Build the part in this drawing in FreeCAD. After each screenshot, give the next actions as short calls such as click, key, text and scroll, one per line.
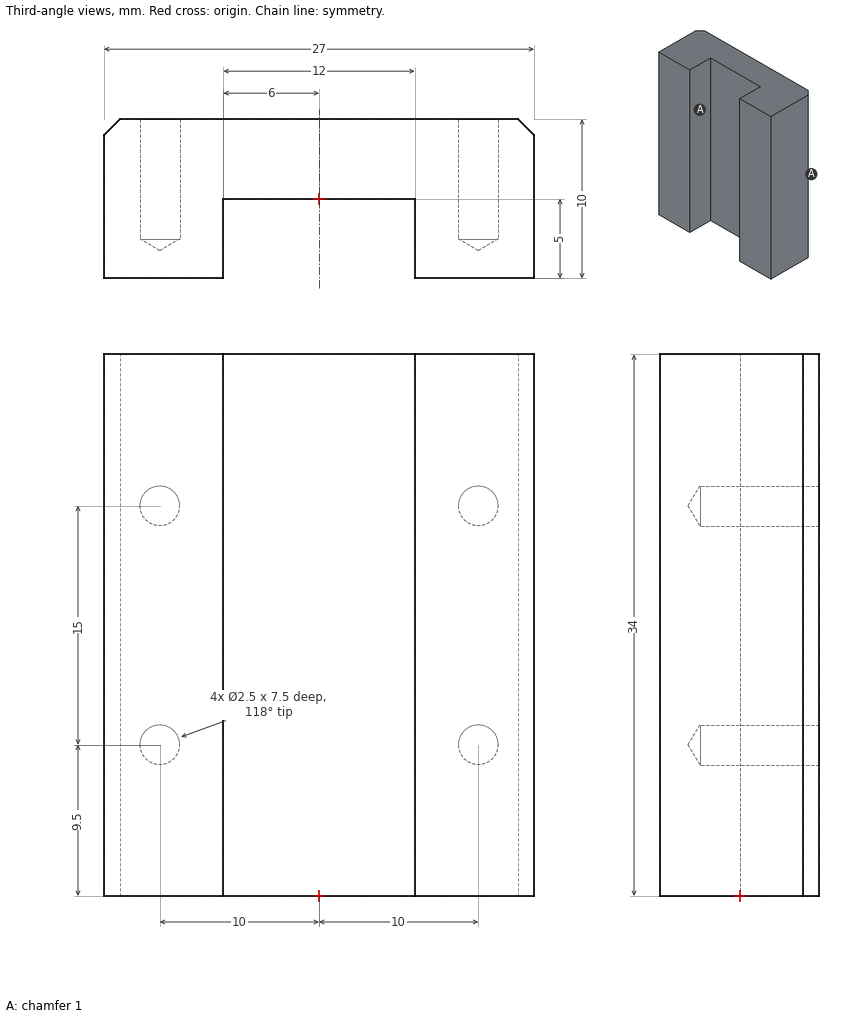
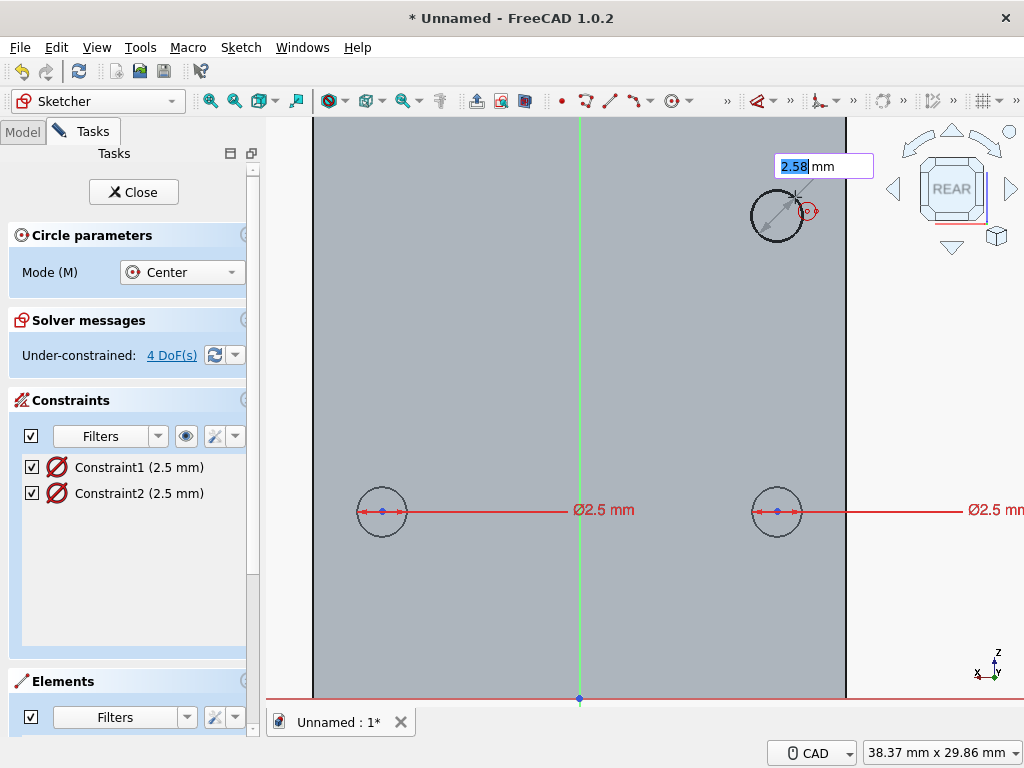
text(2.5)
key(Return)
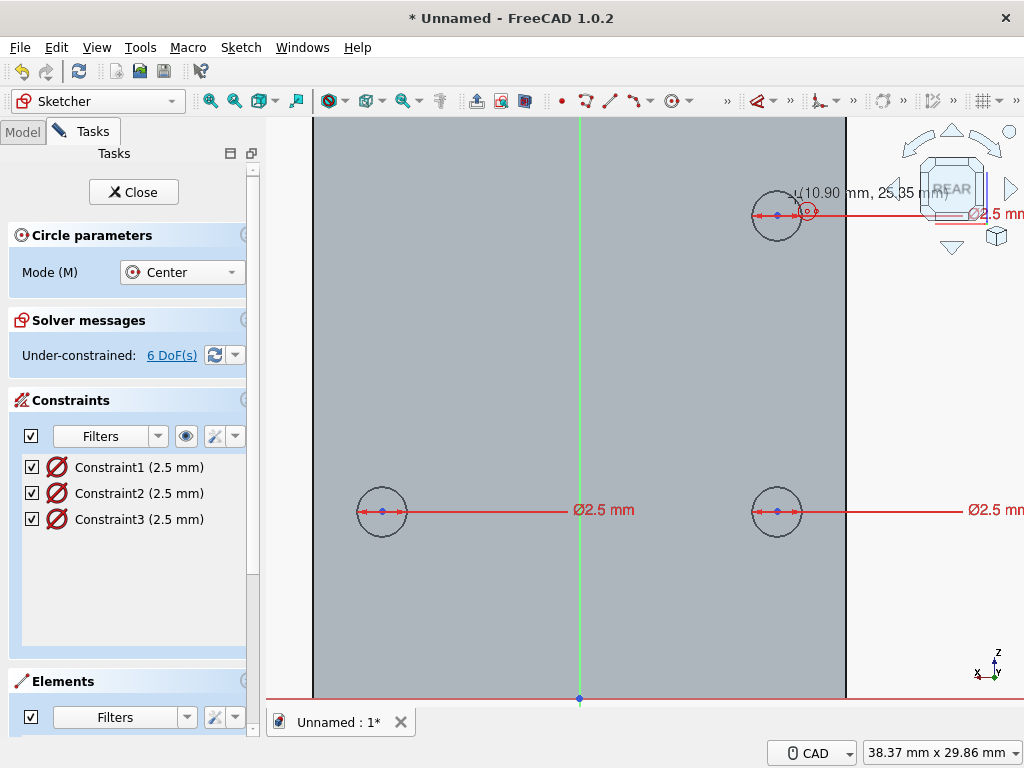
click(382, 215)
move(400, 197)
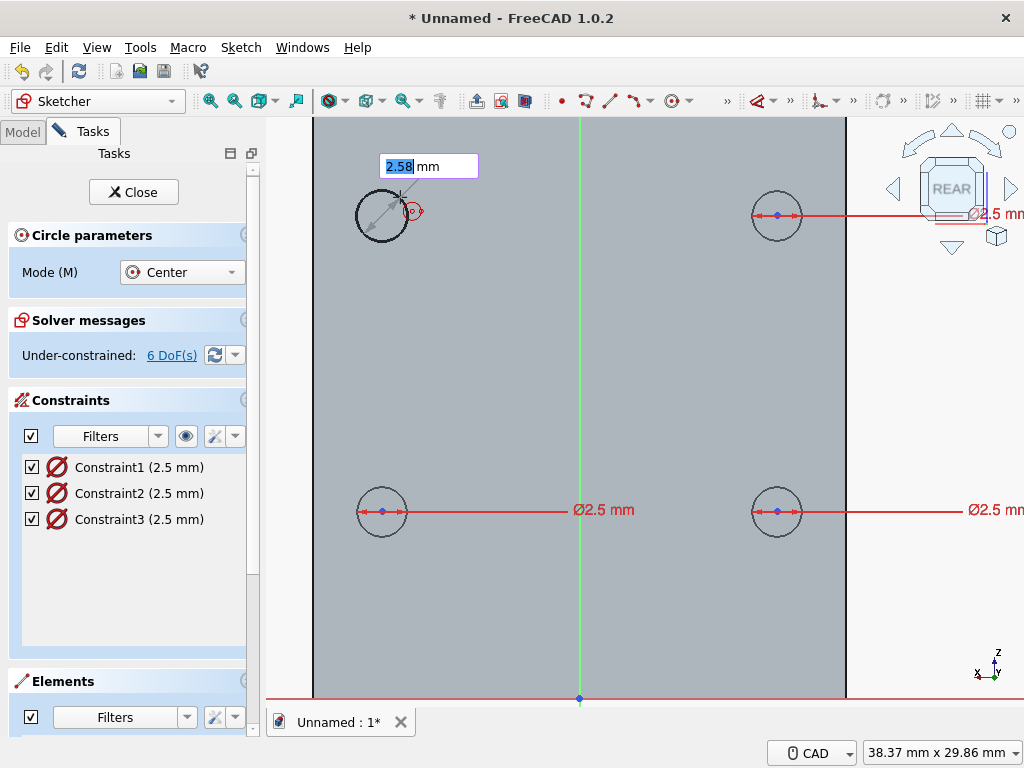
text(2.5)
key(Return)
key(Escape)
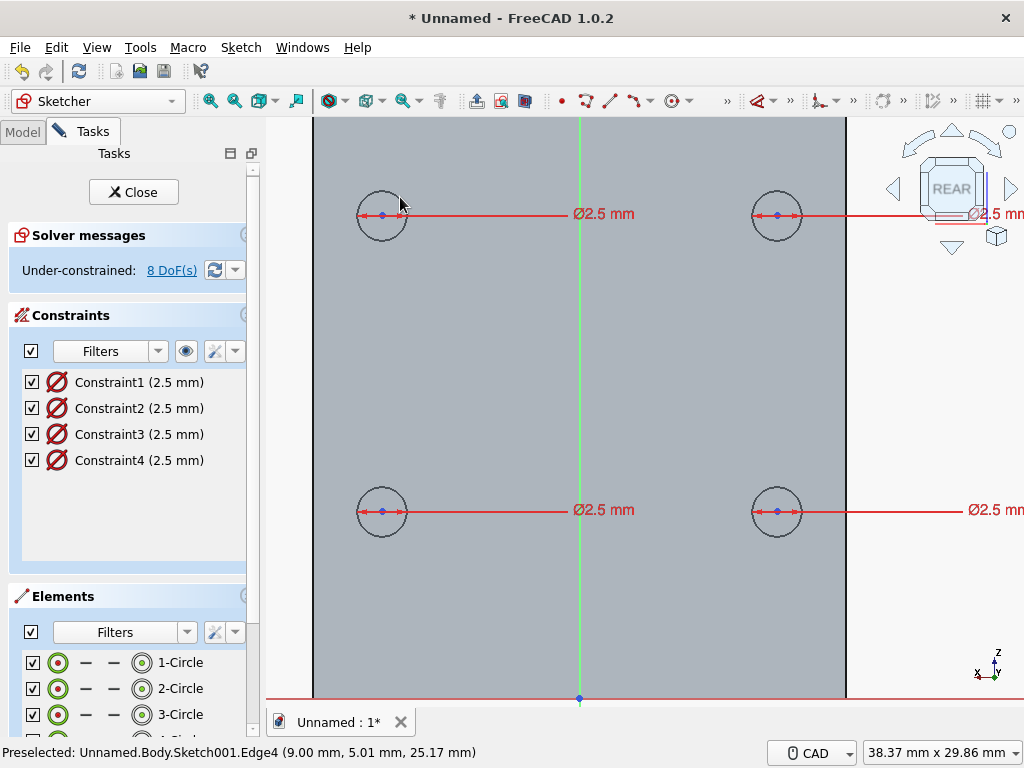
click(777, 512)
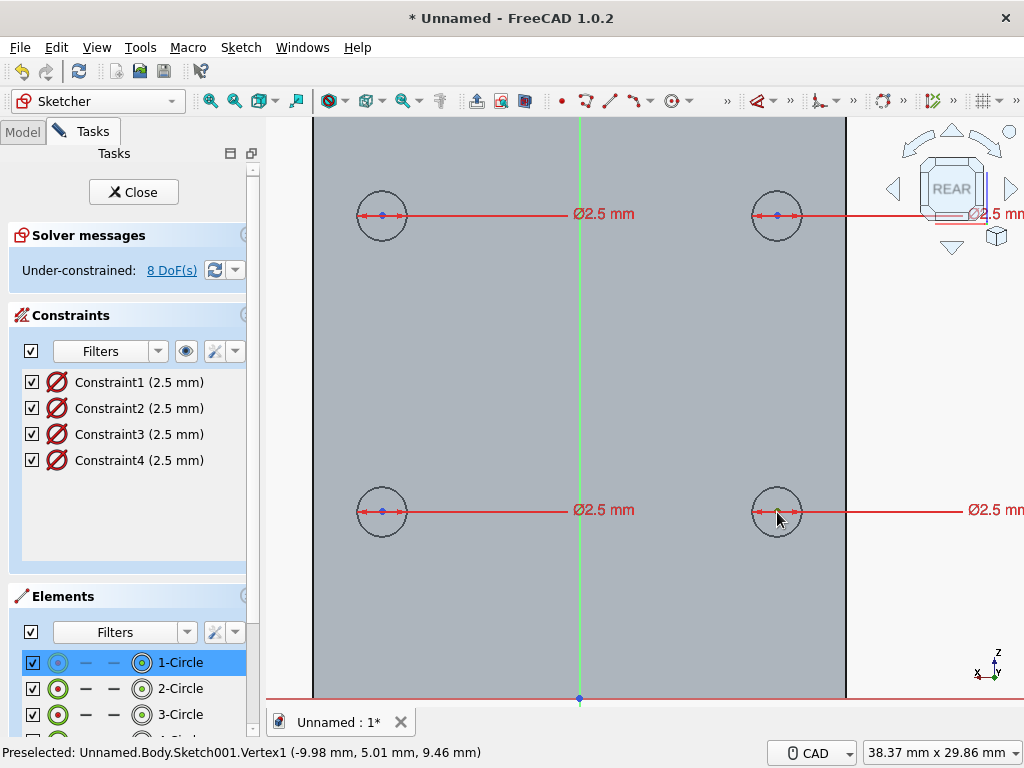
click(382, 512)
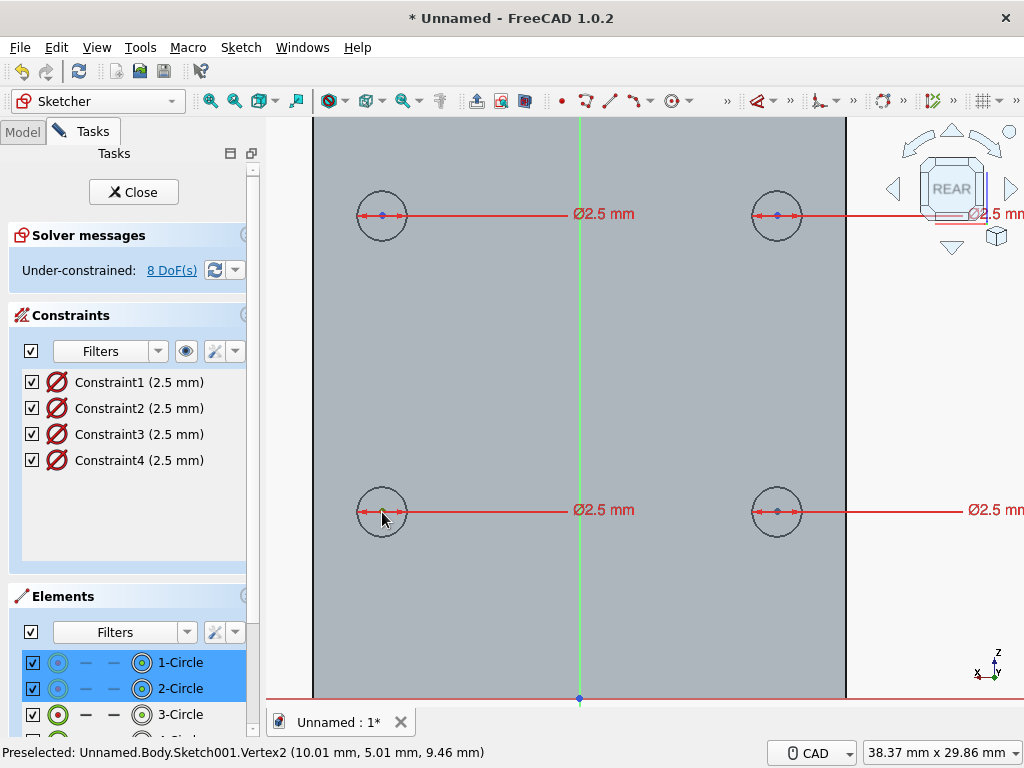
key(h)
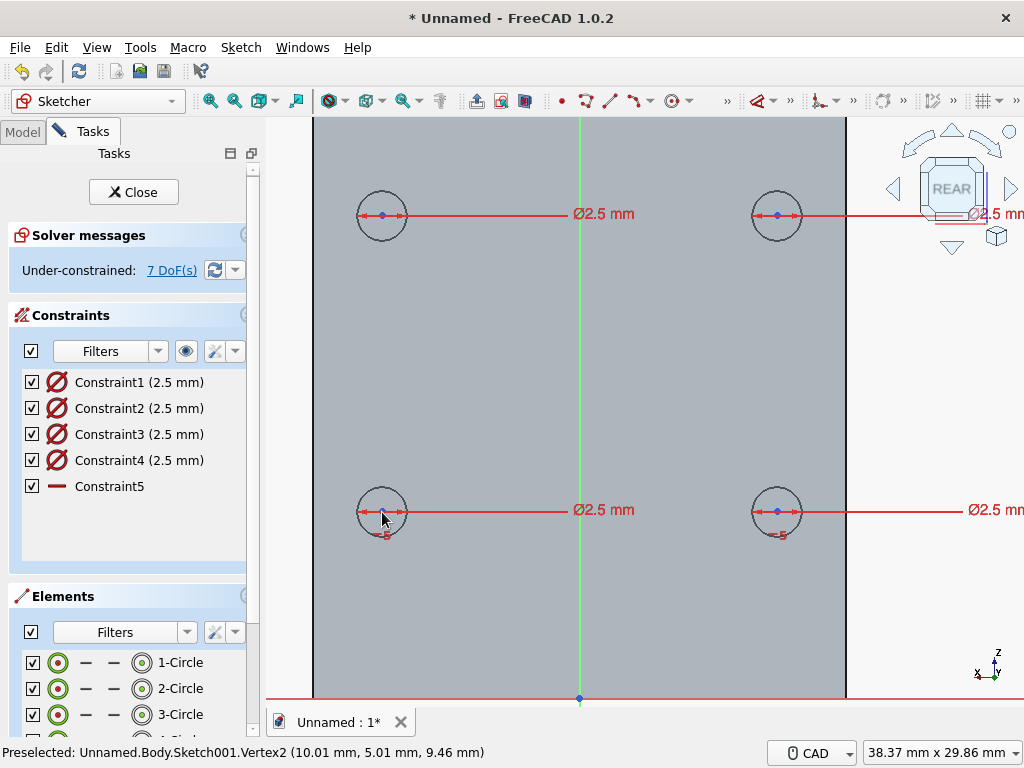
click(777, 512)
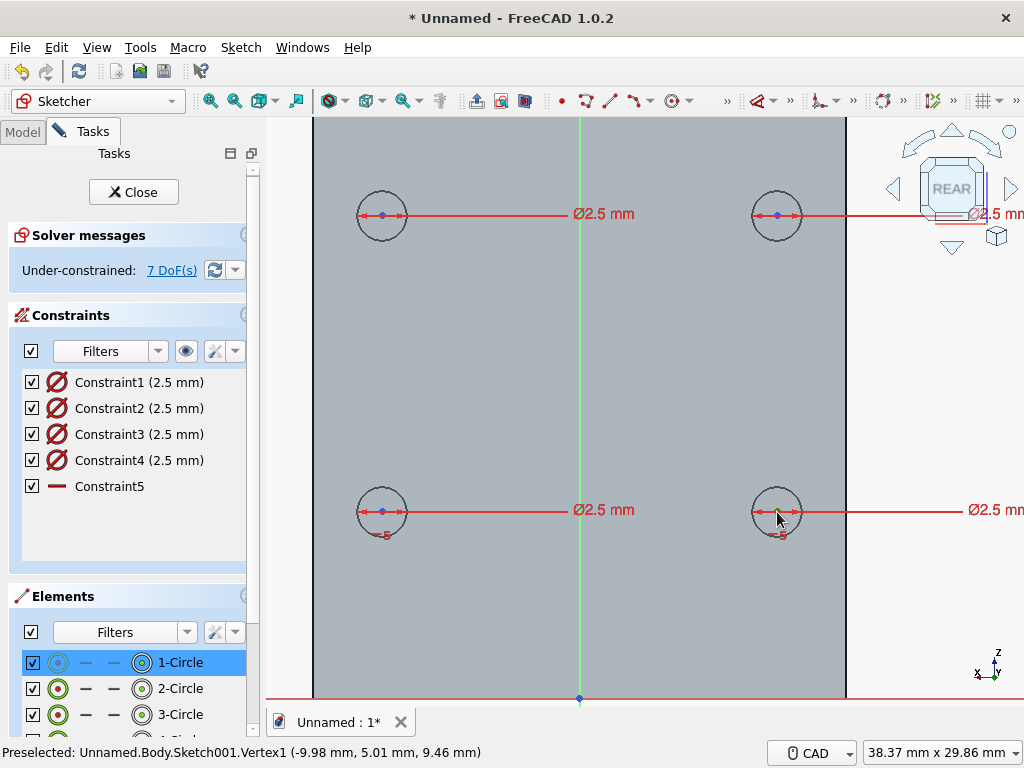
click(777, 216)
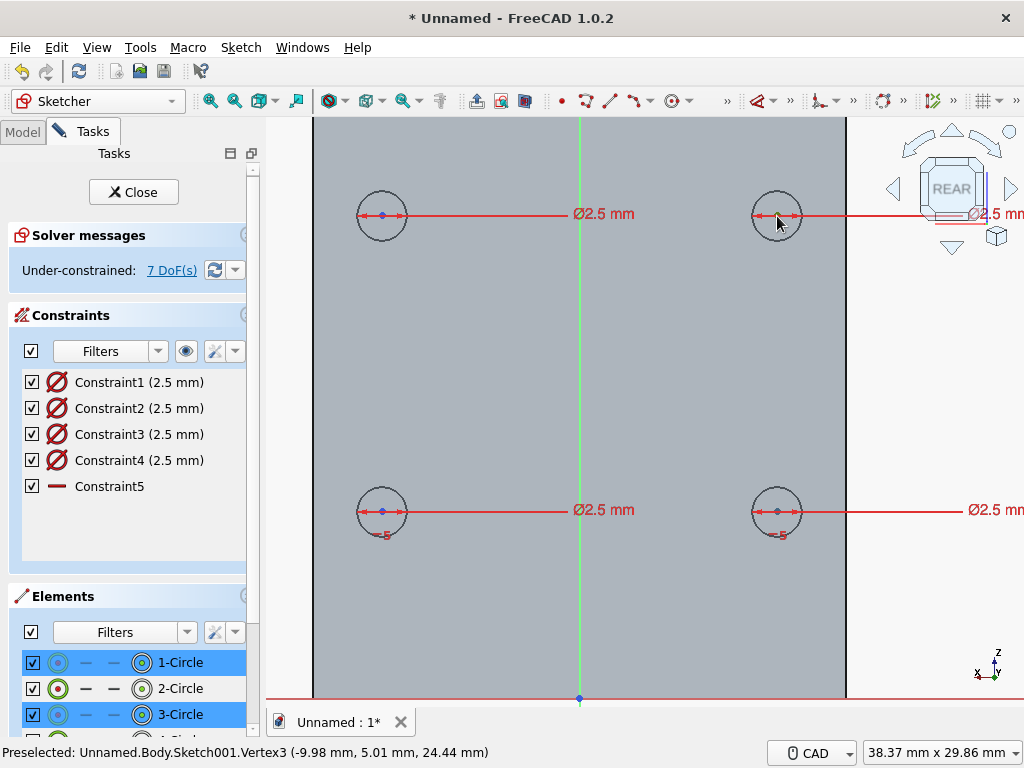
key(v)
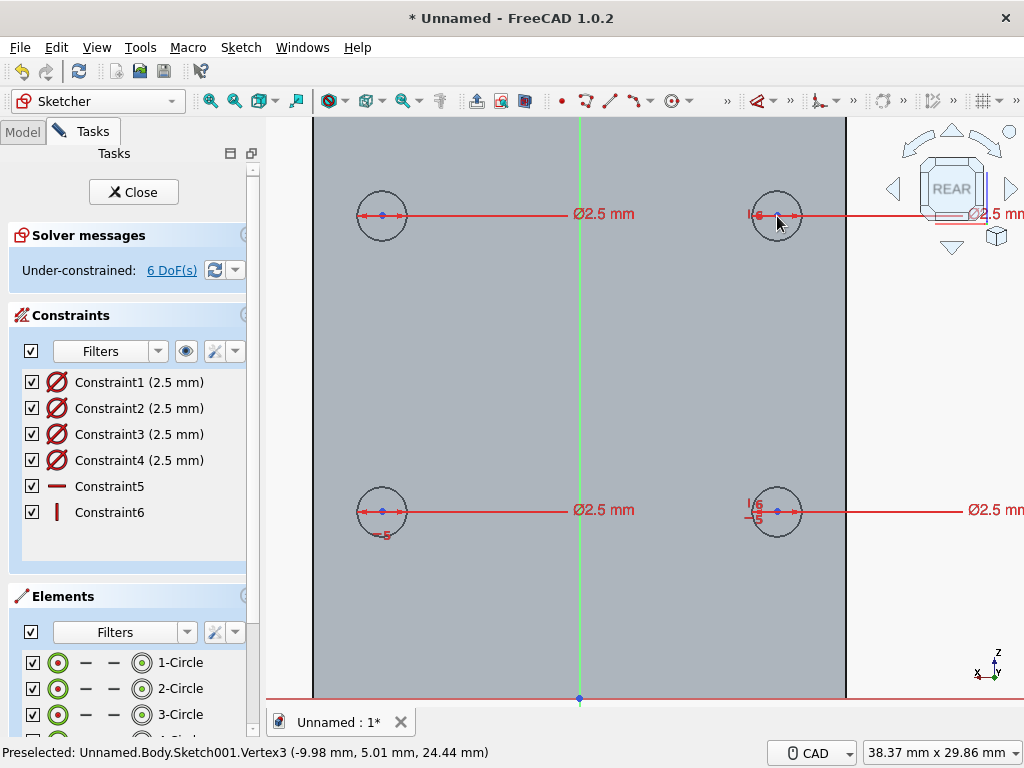
click(382, 512)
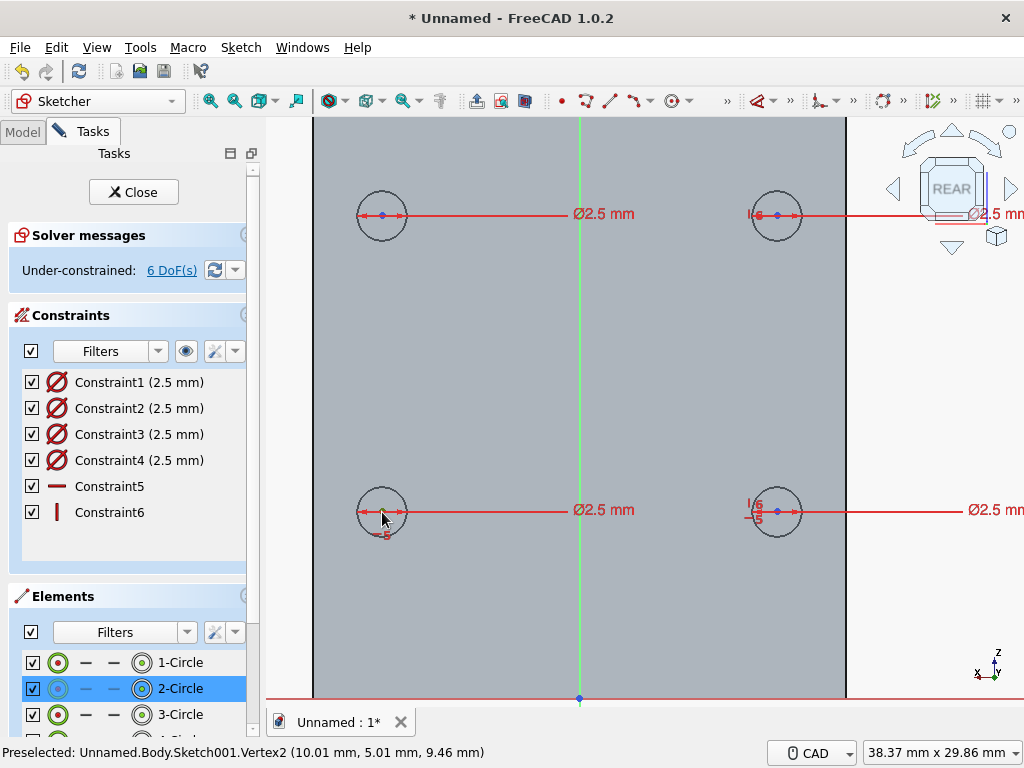
click(382, 216)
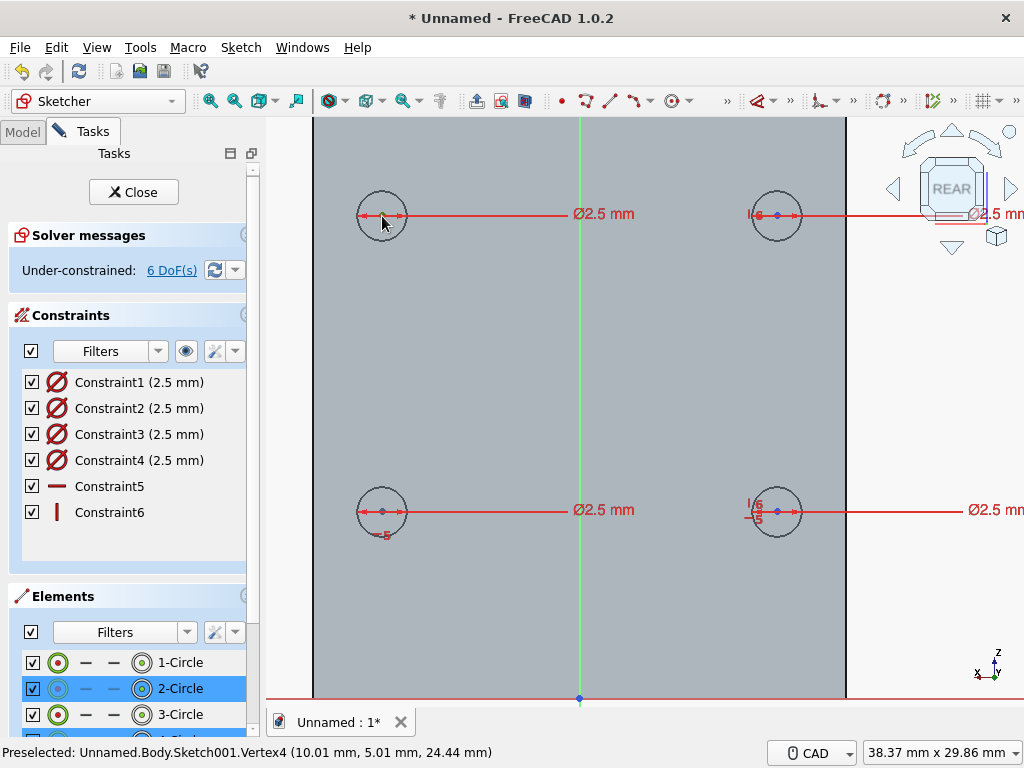
key(v)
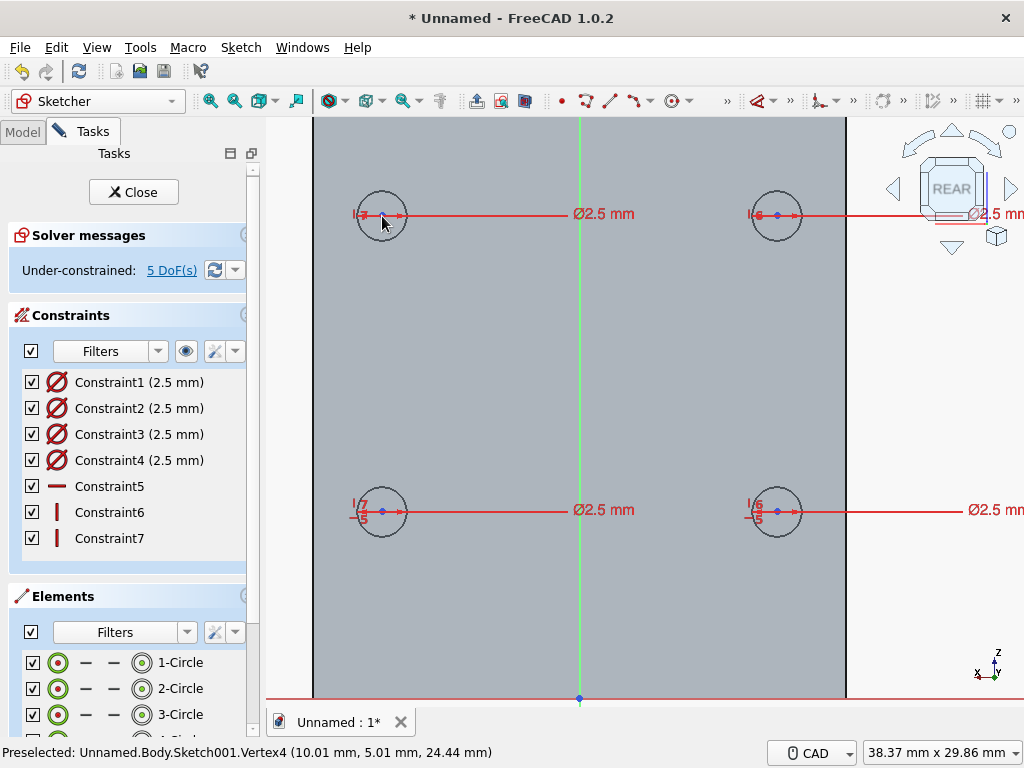
click(777, 216)